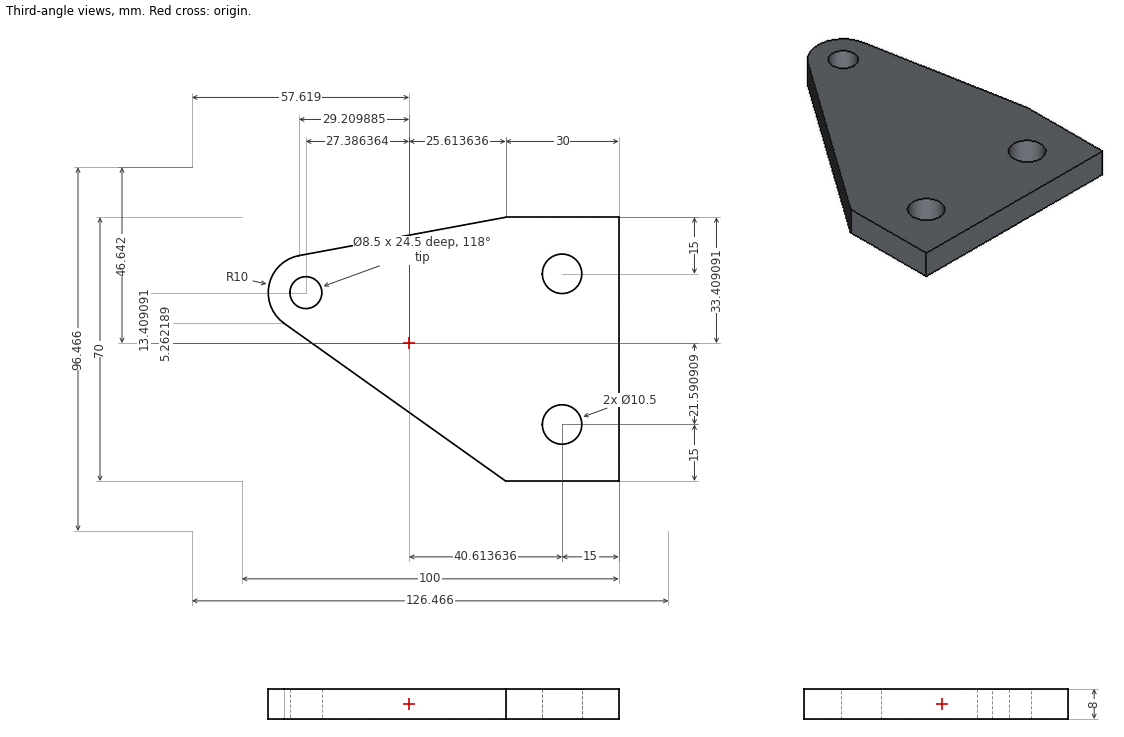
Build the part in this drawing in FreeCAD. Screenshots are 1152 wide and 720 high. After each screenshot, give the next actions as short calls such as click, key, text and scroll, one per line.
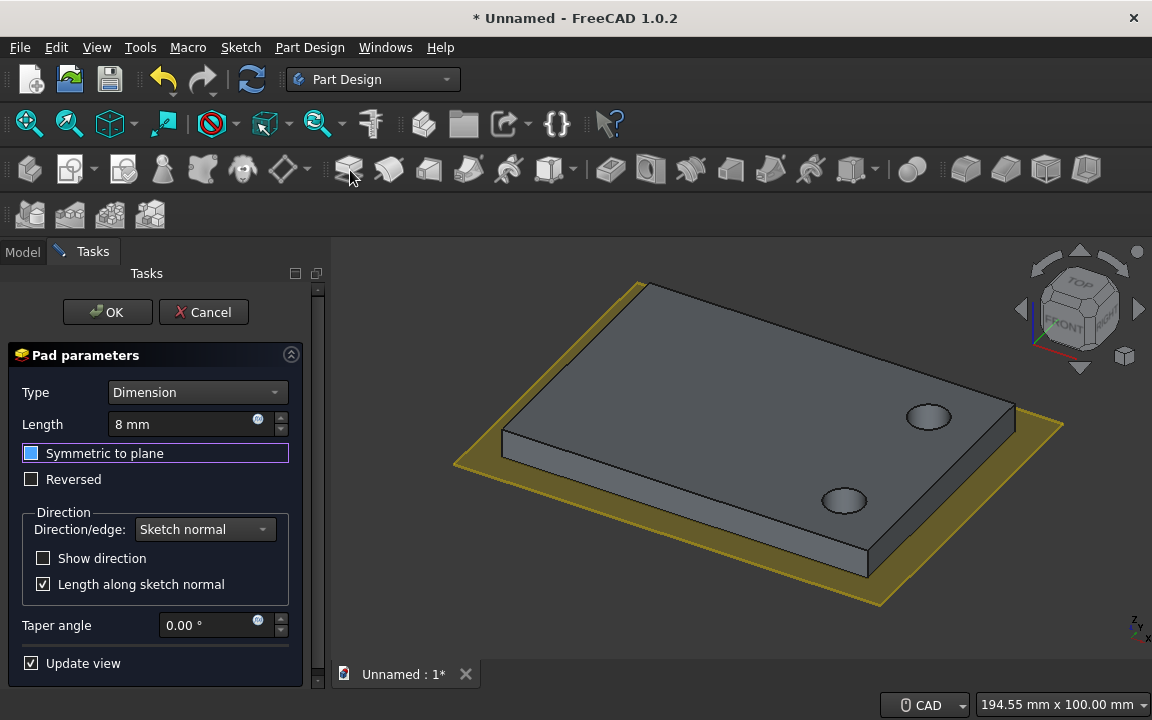
click(30, 479)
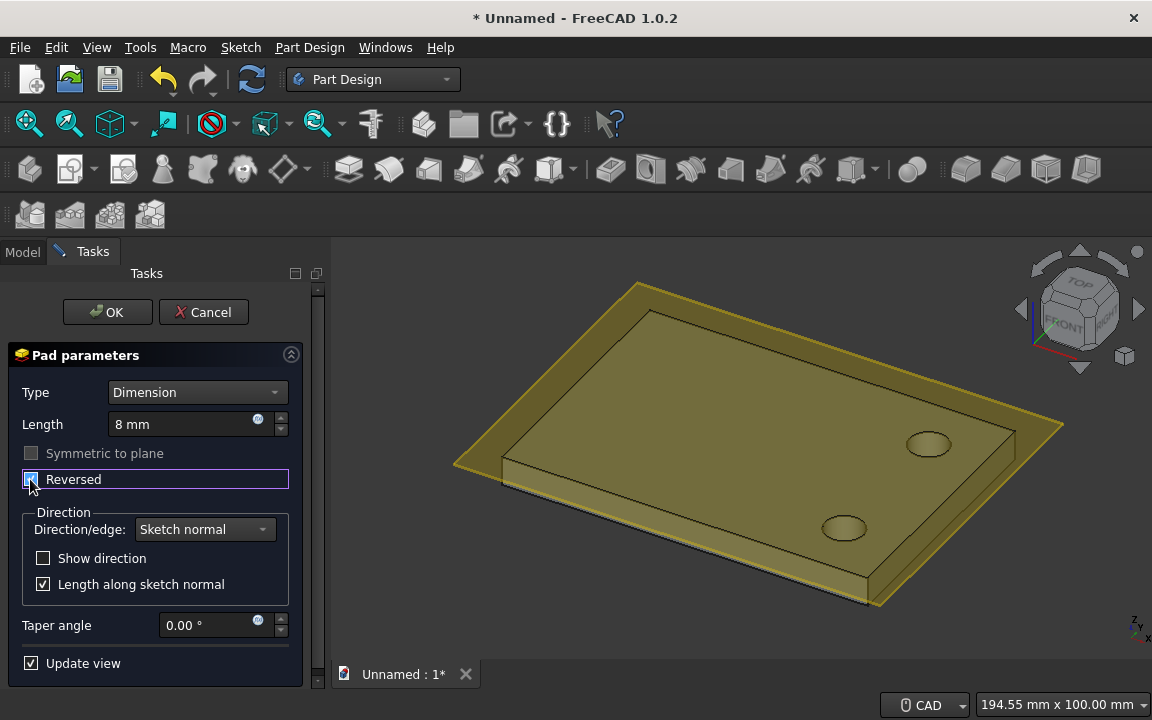
click(108, 312)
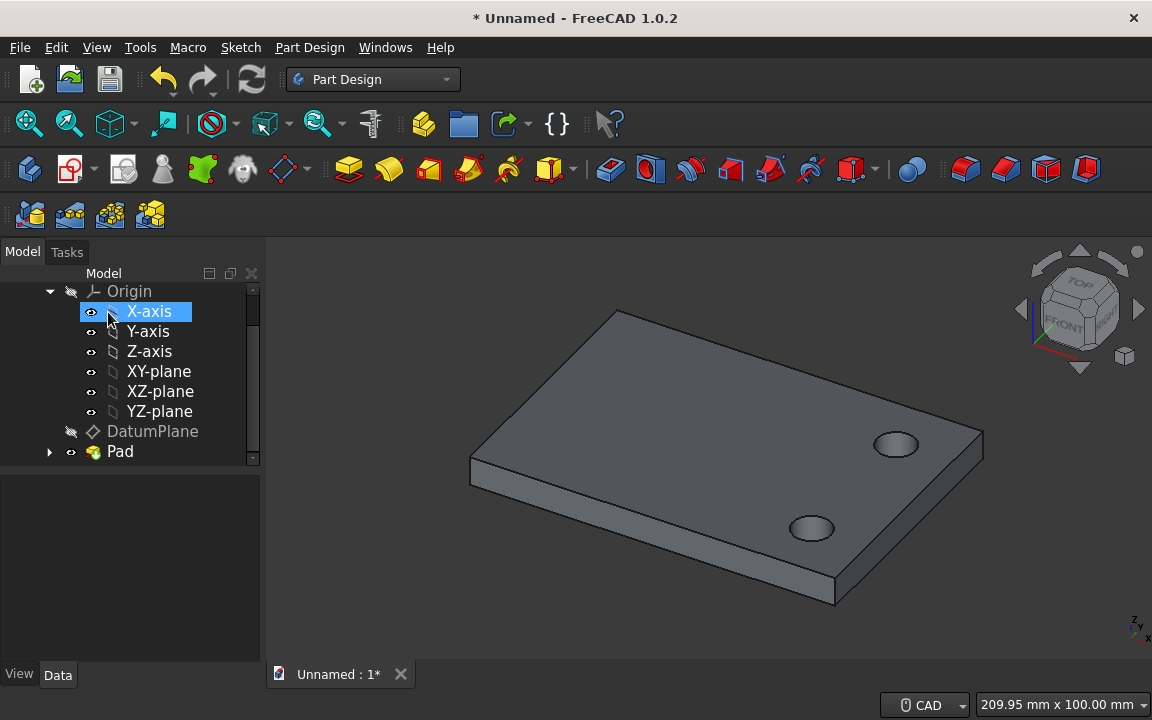
click(726, 443)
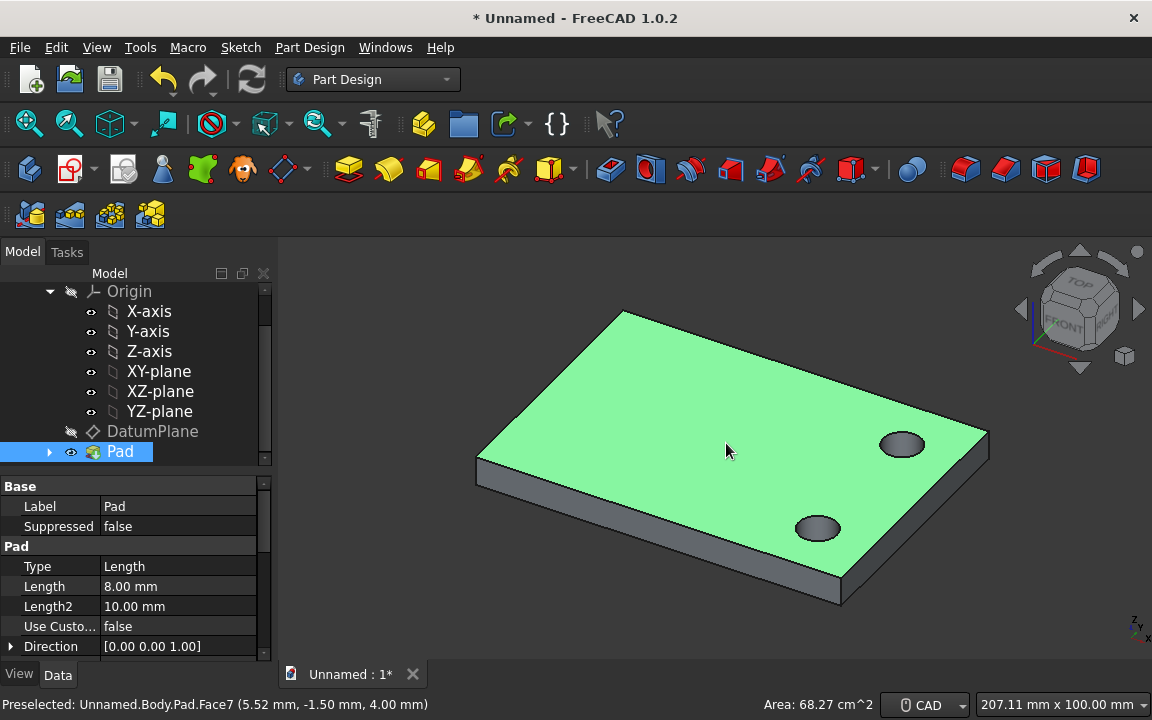
click(70, 170)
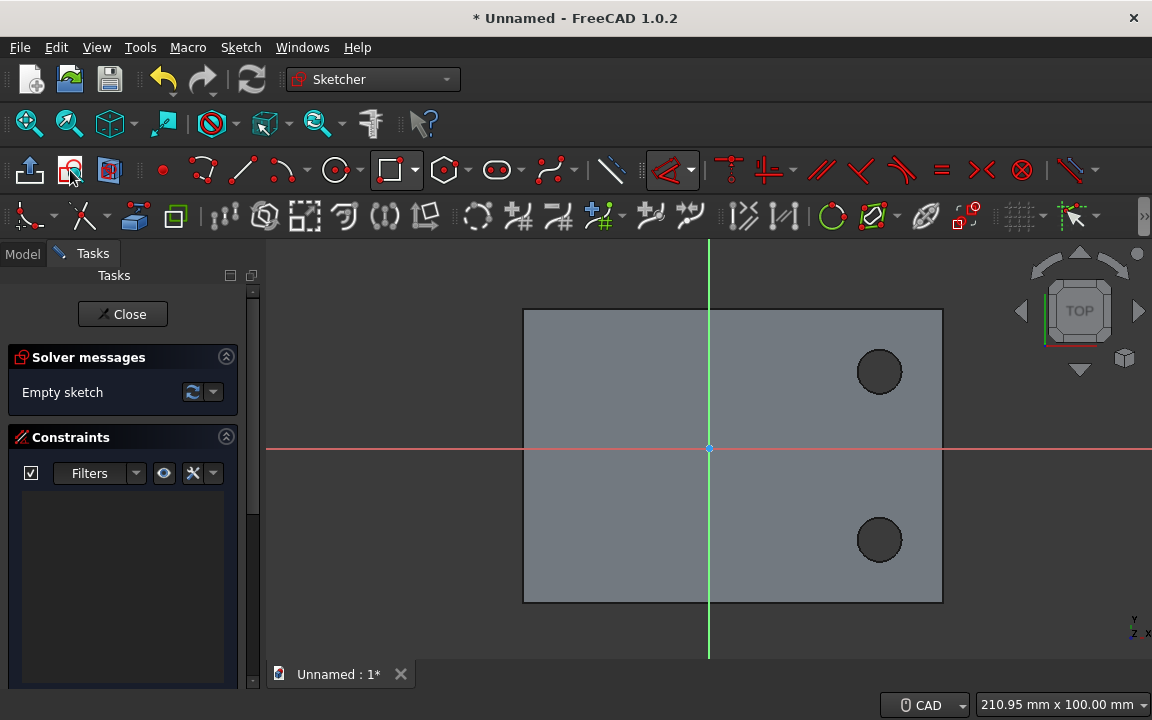
scroll(453, 435, down, 2)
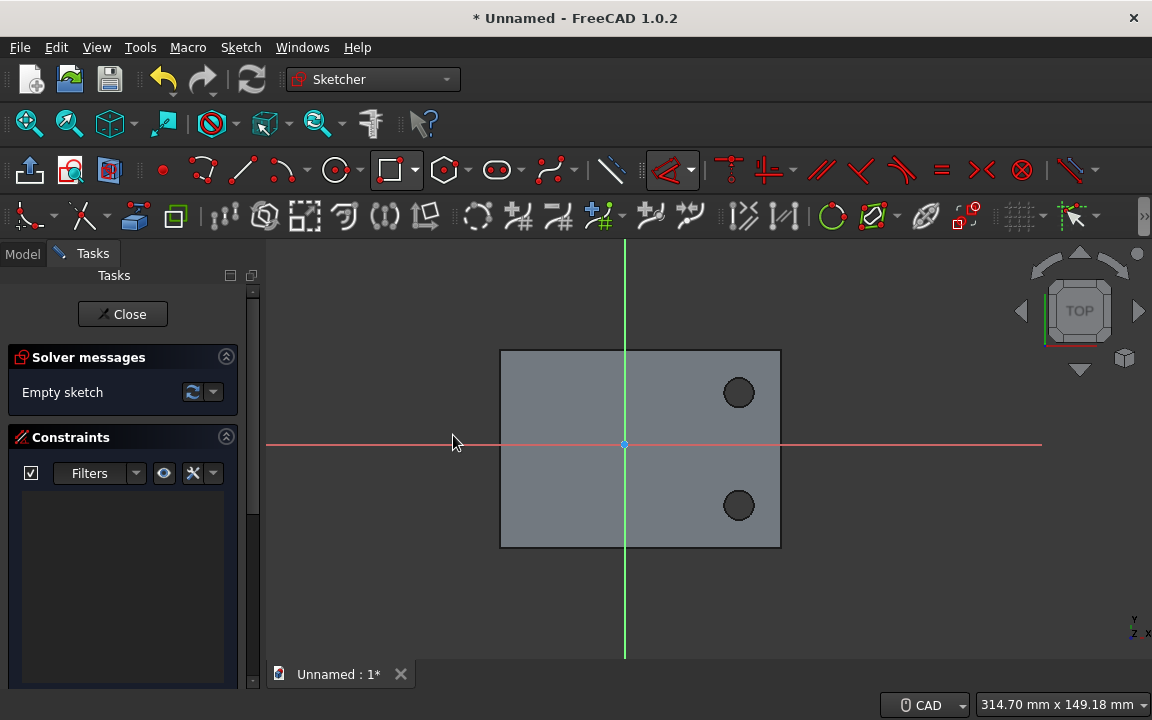
click(390, 170)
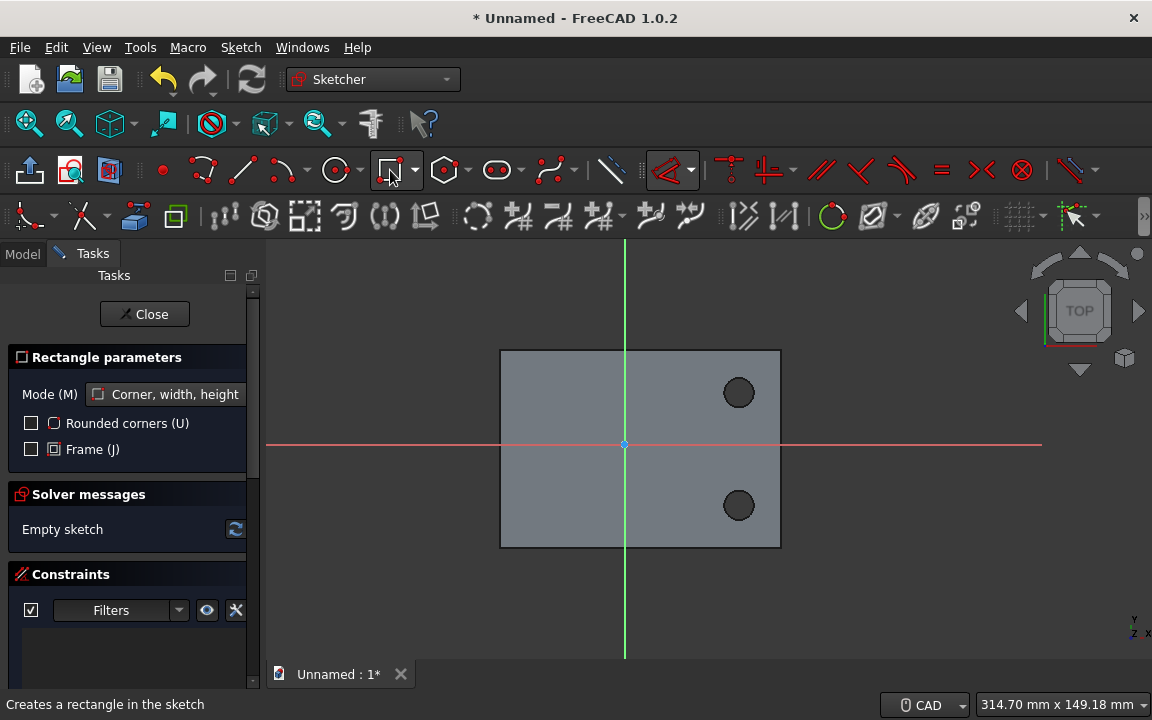
click(462, 313)
click(818, 585)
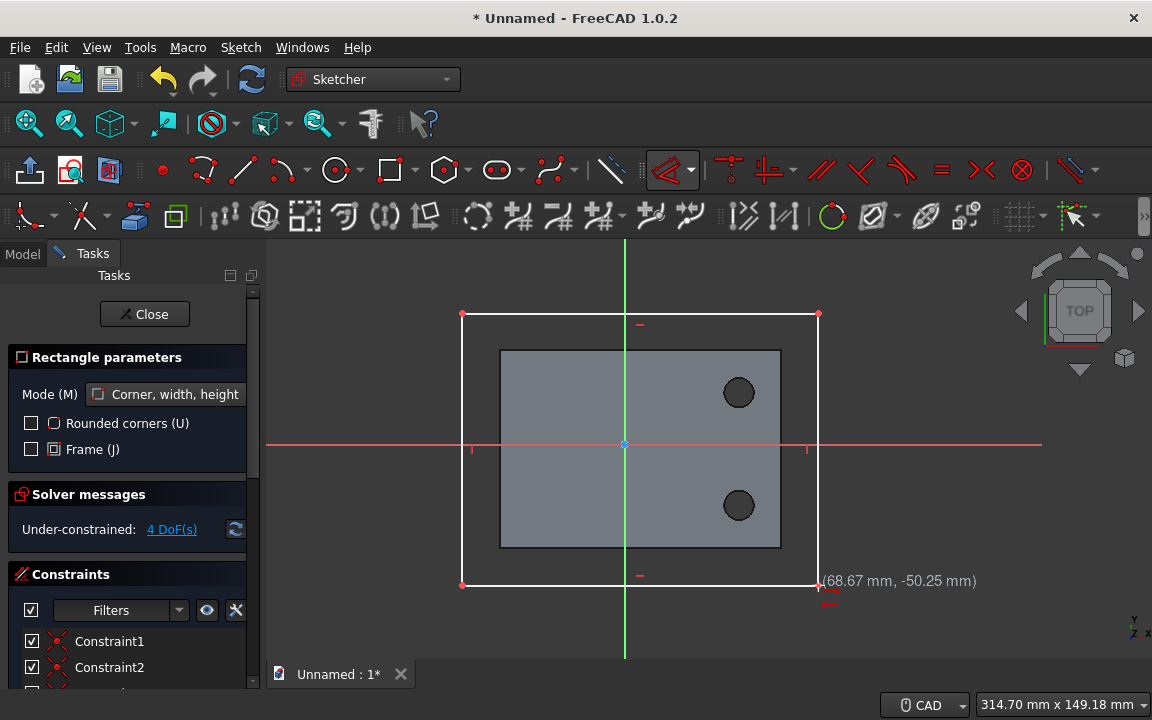
key(g)
key(m)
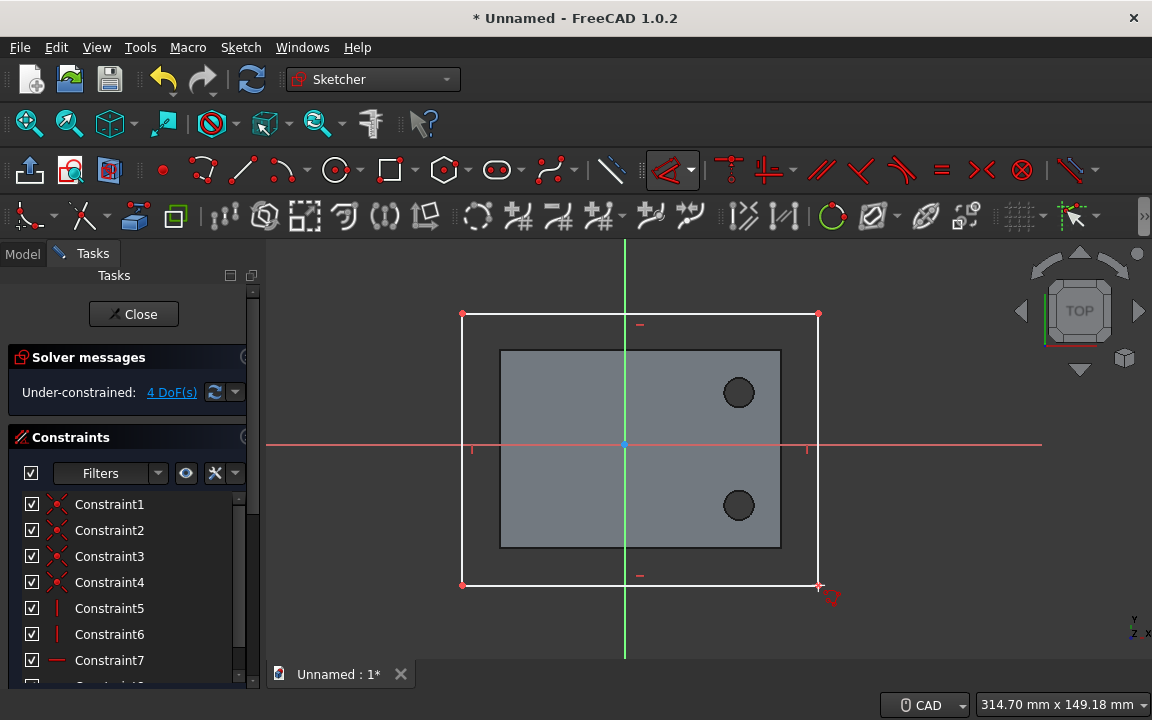
click(542, 379)
click(697, 350)
click(781, 350)
click(781, 548)
click(697, 548)
click(531, 430)
right_click(531, 430)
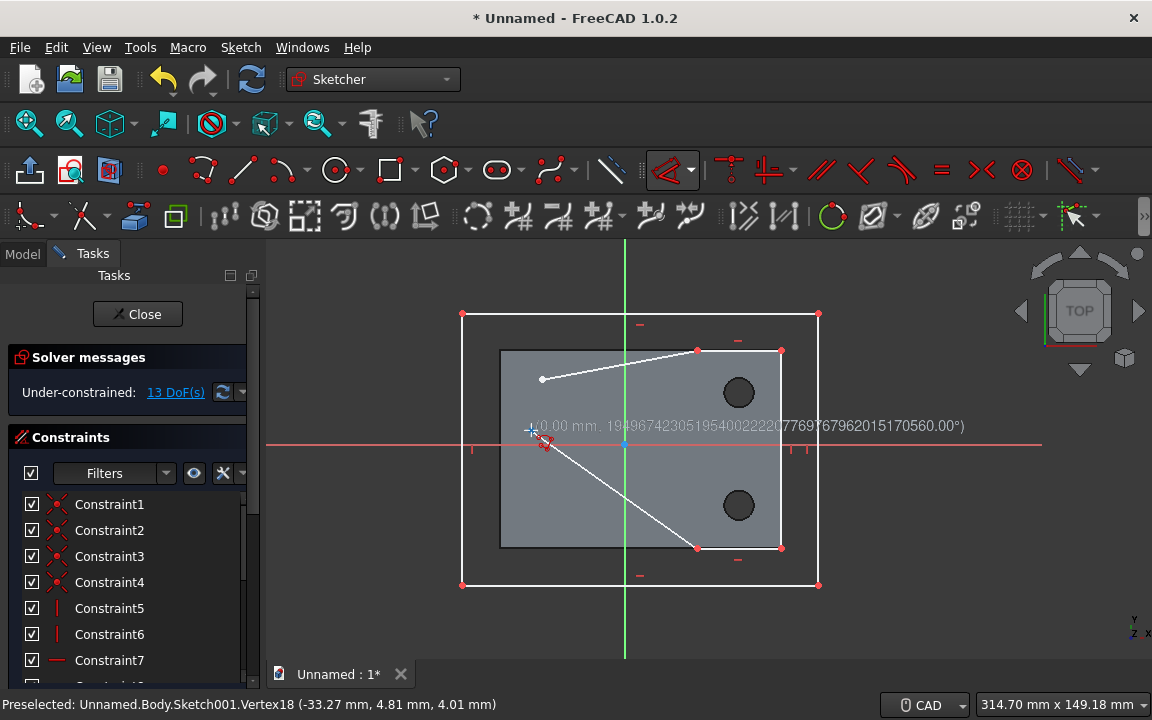
key(g)
key(3)
key(a)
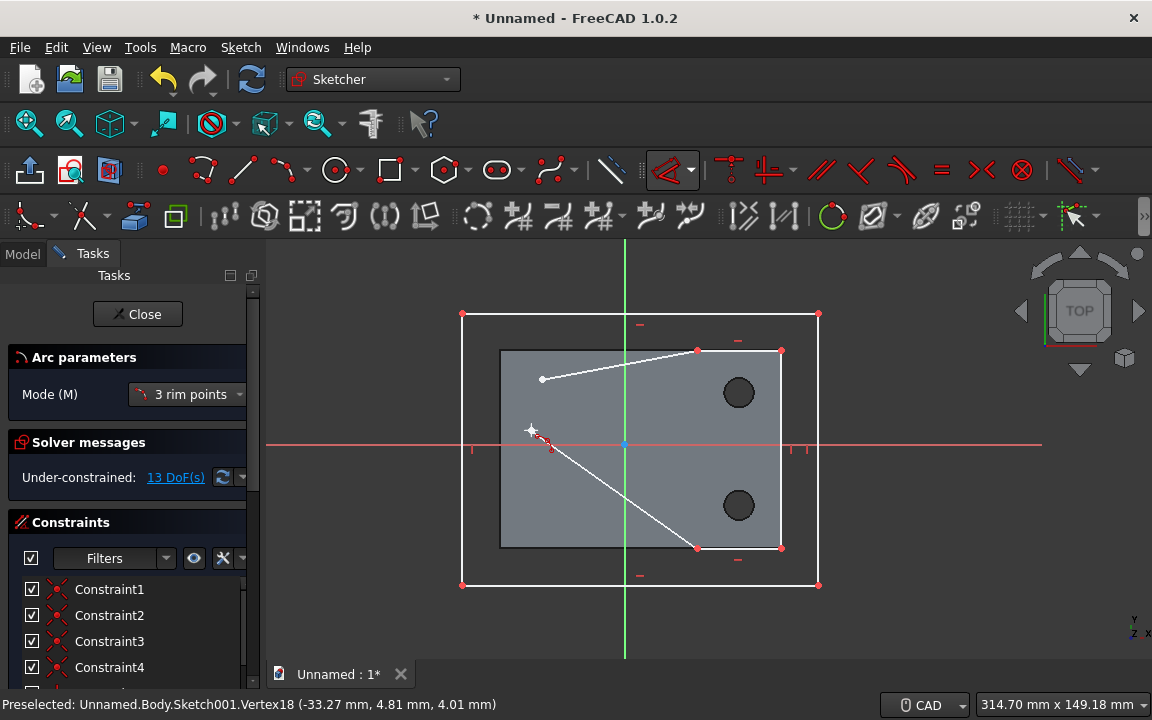
click(531, 431)
click(542, 380)
click(520, 401)
key(Escape)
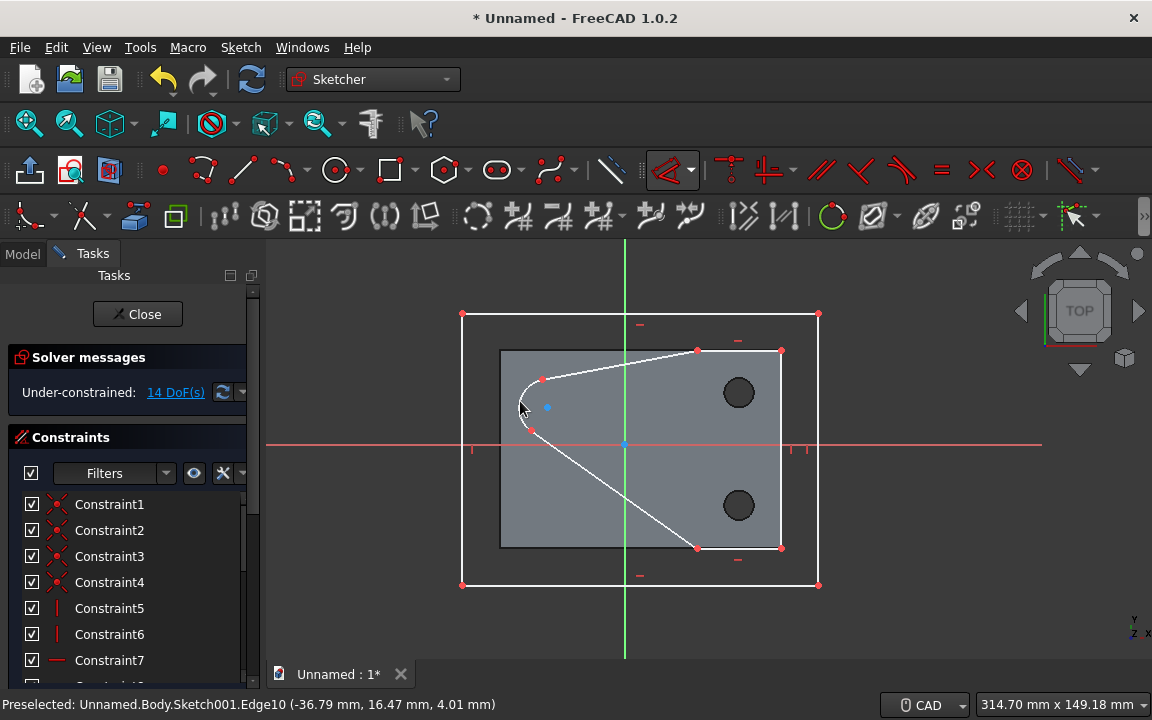
click(589, 371)